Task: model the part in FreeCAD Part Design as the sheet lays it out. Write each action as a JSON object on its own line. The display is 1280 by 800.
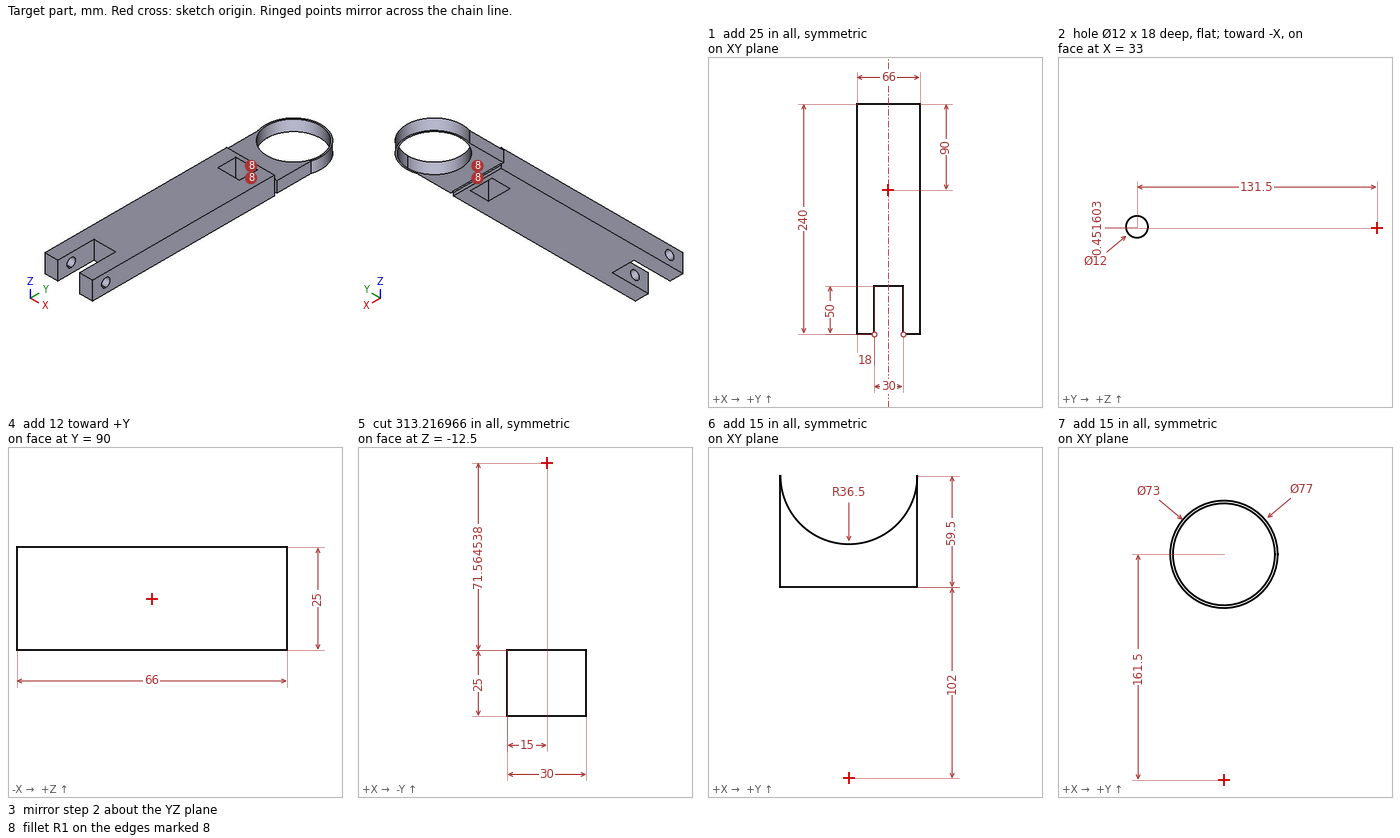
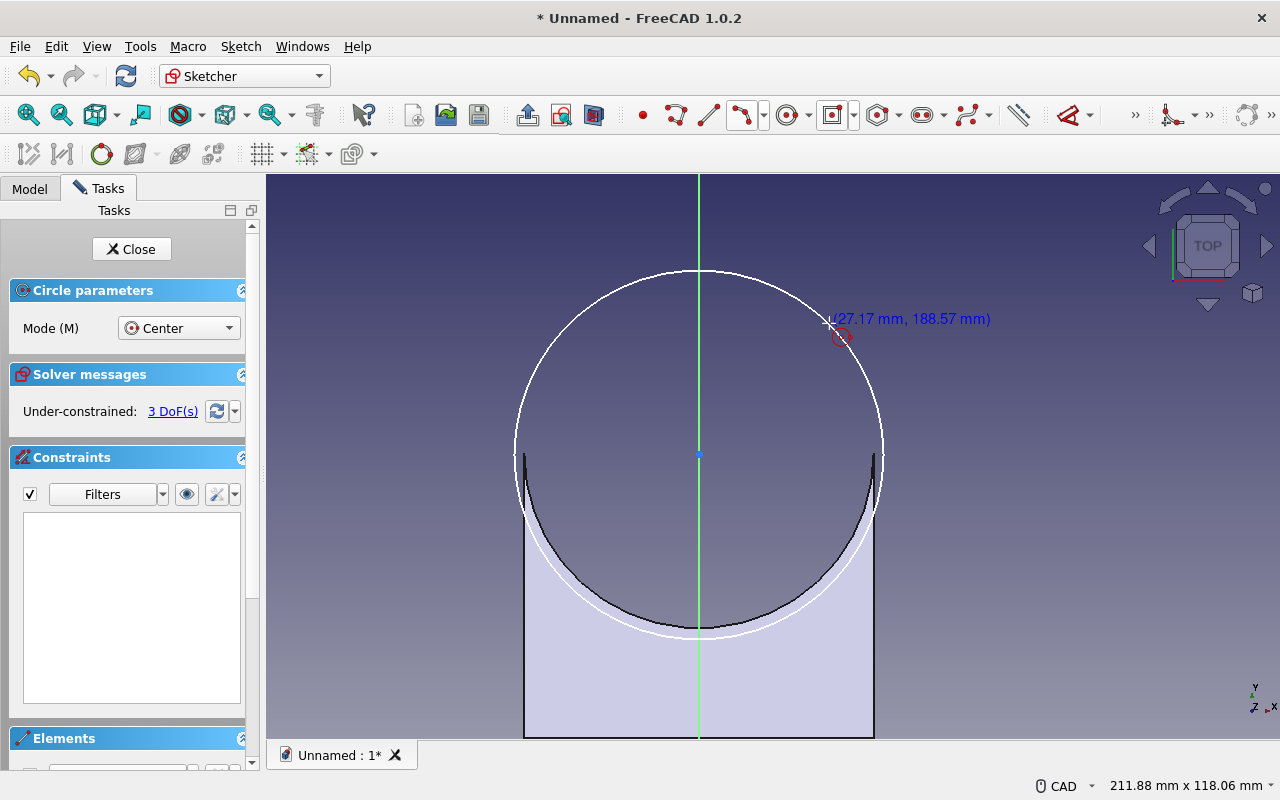
{"action": "left_click", "coordinate": [699, 455]}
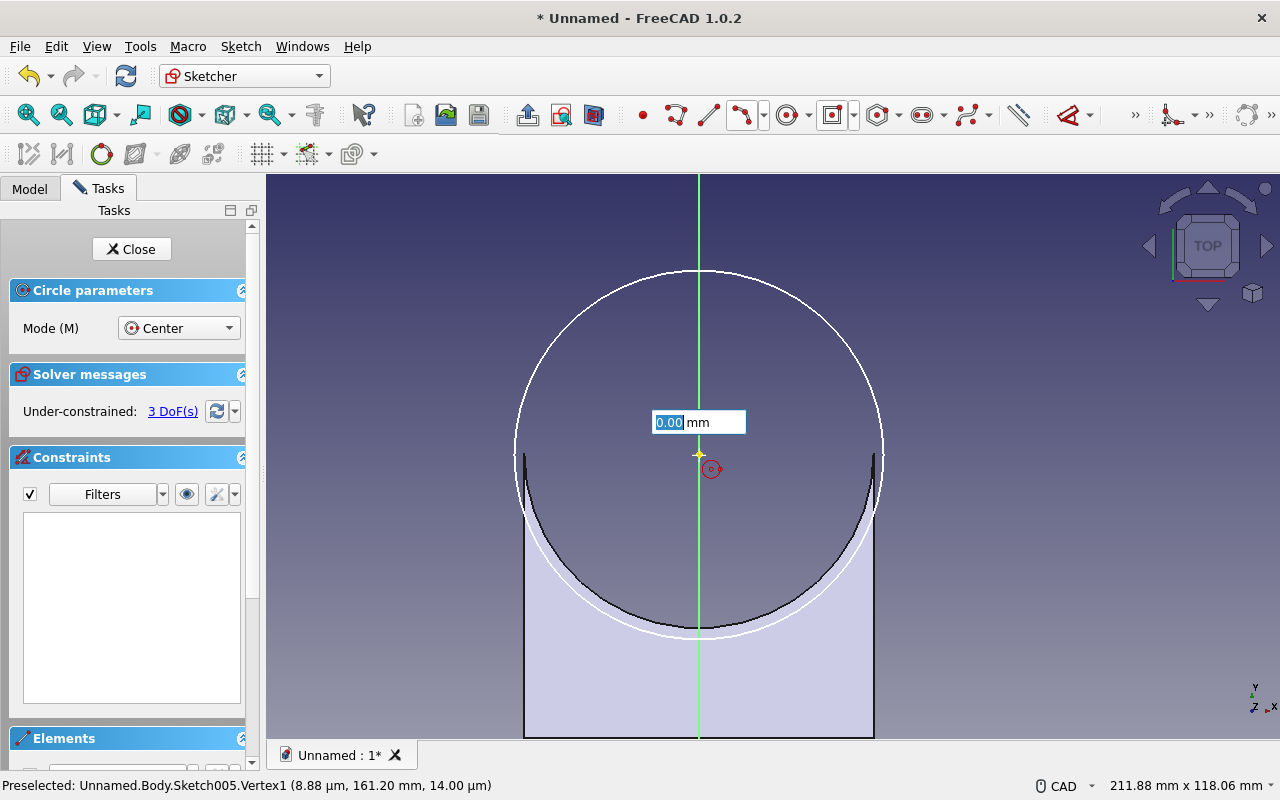
{"action": "scroll", "coordinate": [759, 289], "scroll_direction": "up", "scroll_amount": 3}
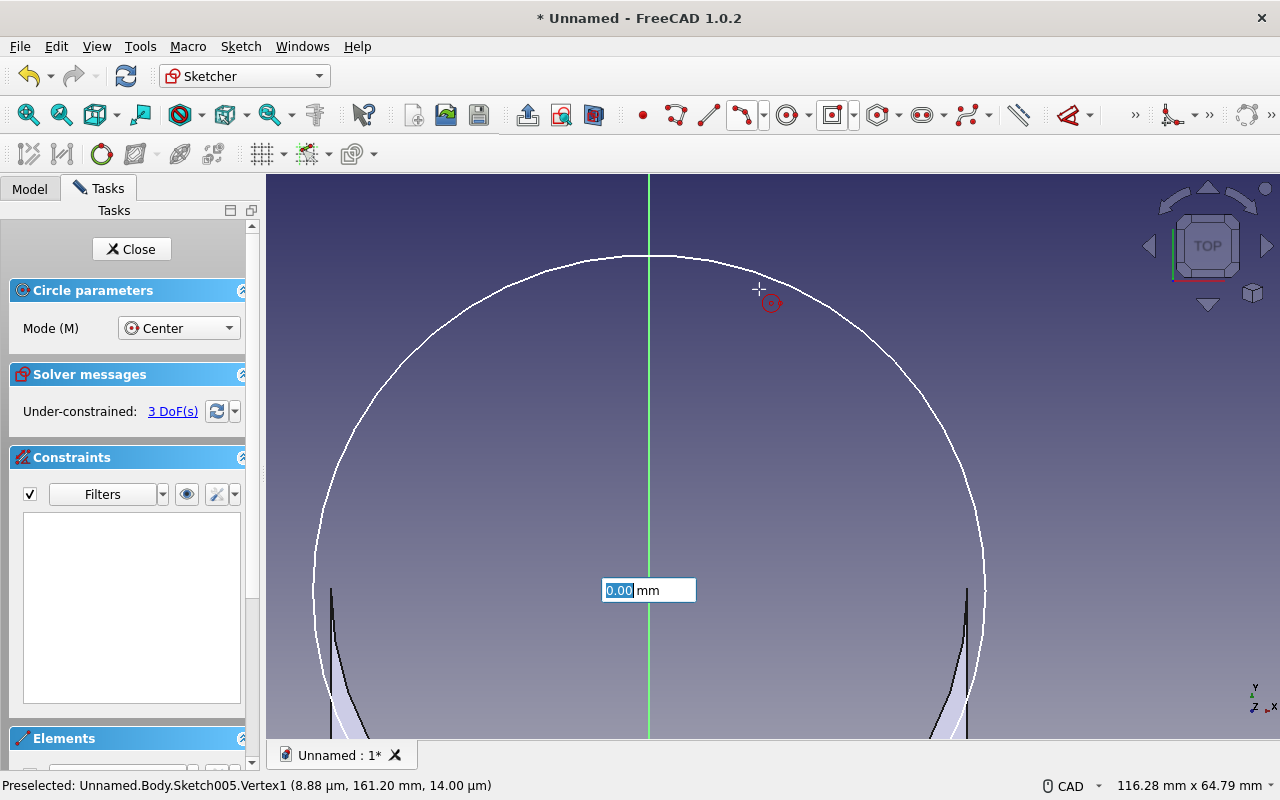
{"action": "left_click", "coordinate": [758, 290]}
{"action": "key", "text": "Escape"}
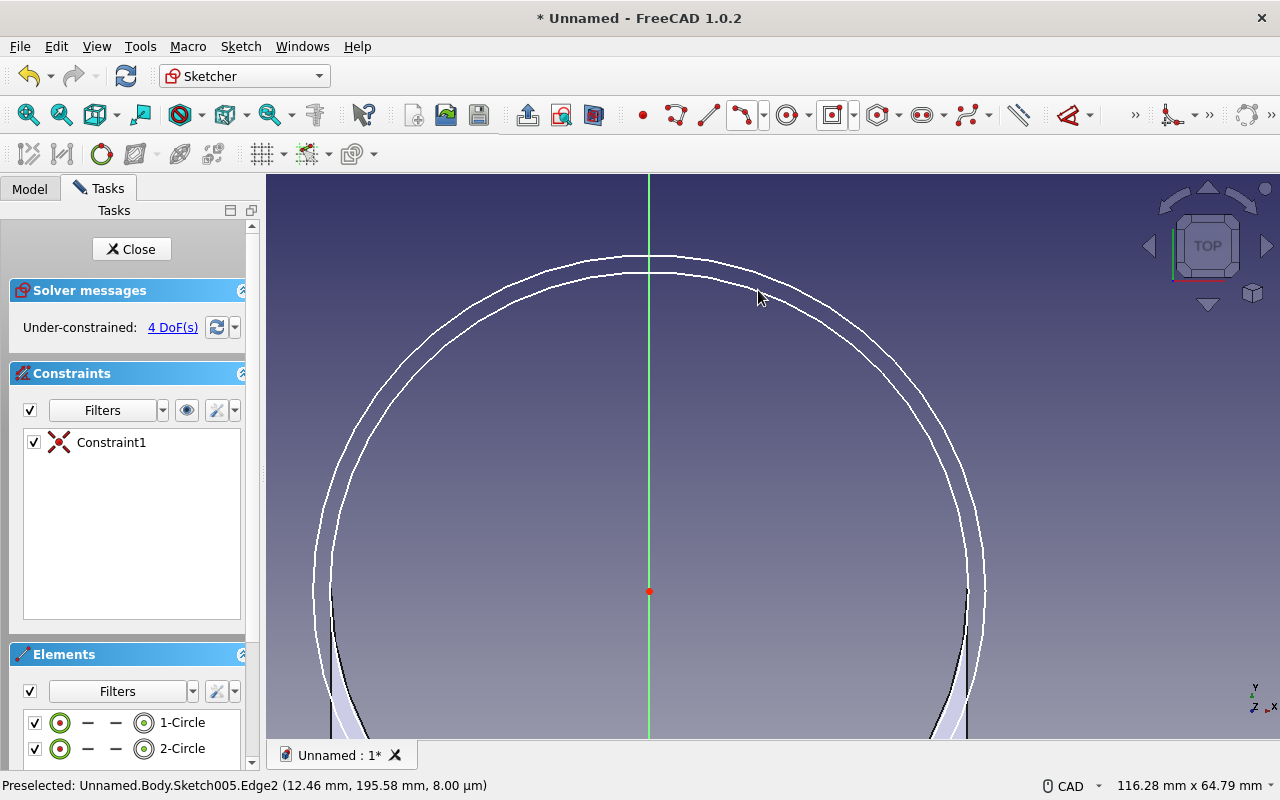
{"action": "left_click", "coordinate": [649, 591]}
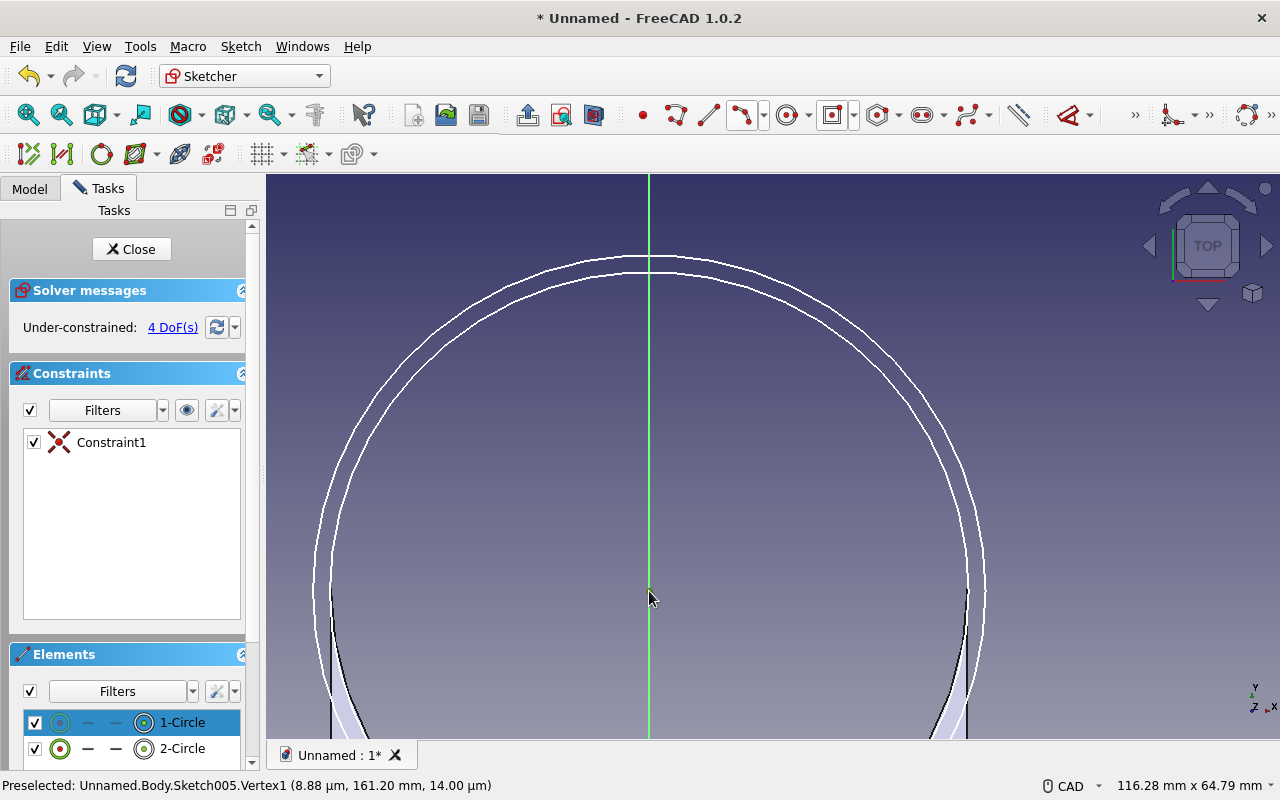
{"action": "left_click", "coordinate": [649, 675]}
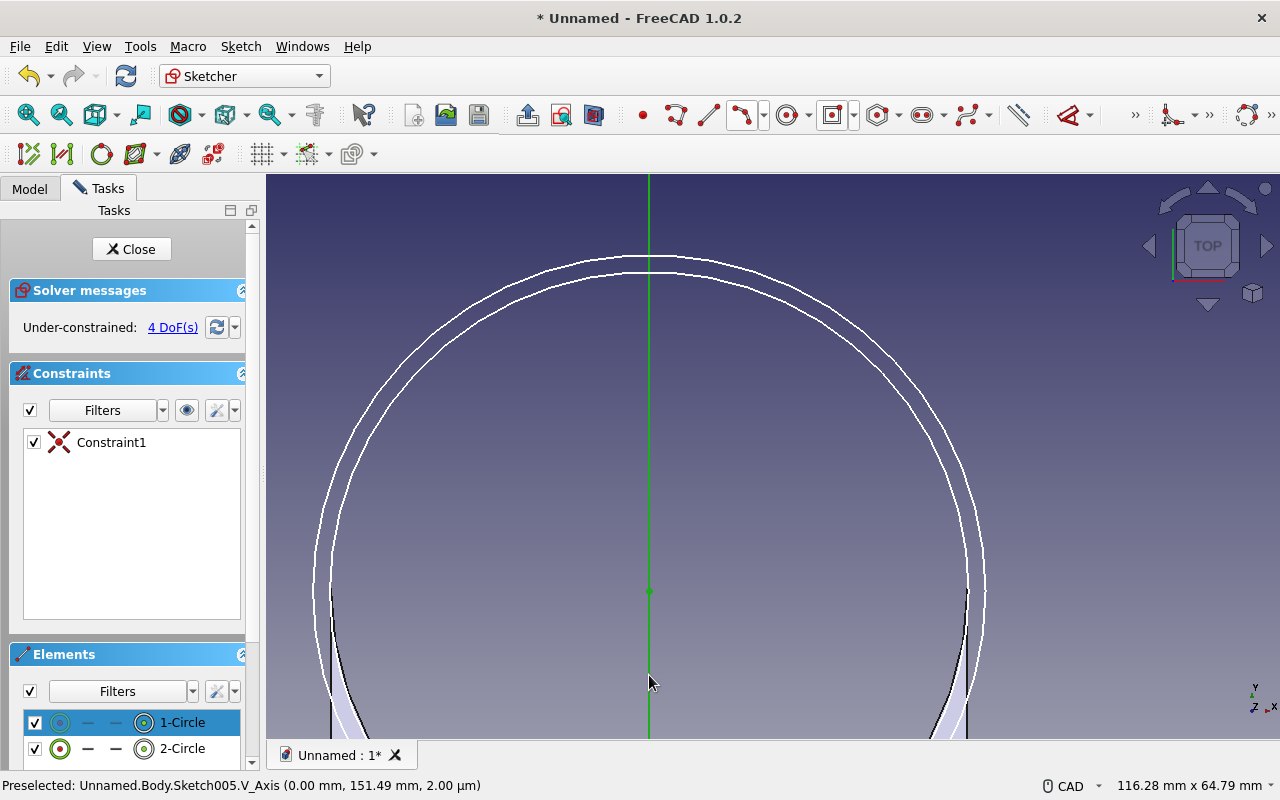
{"action": "key", "text": "c"}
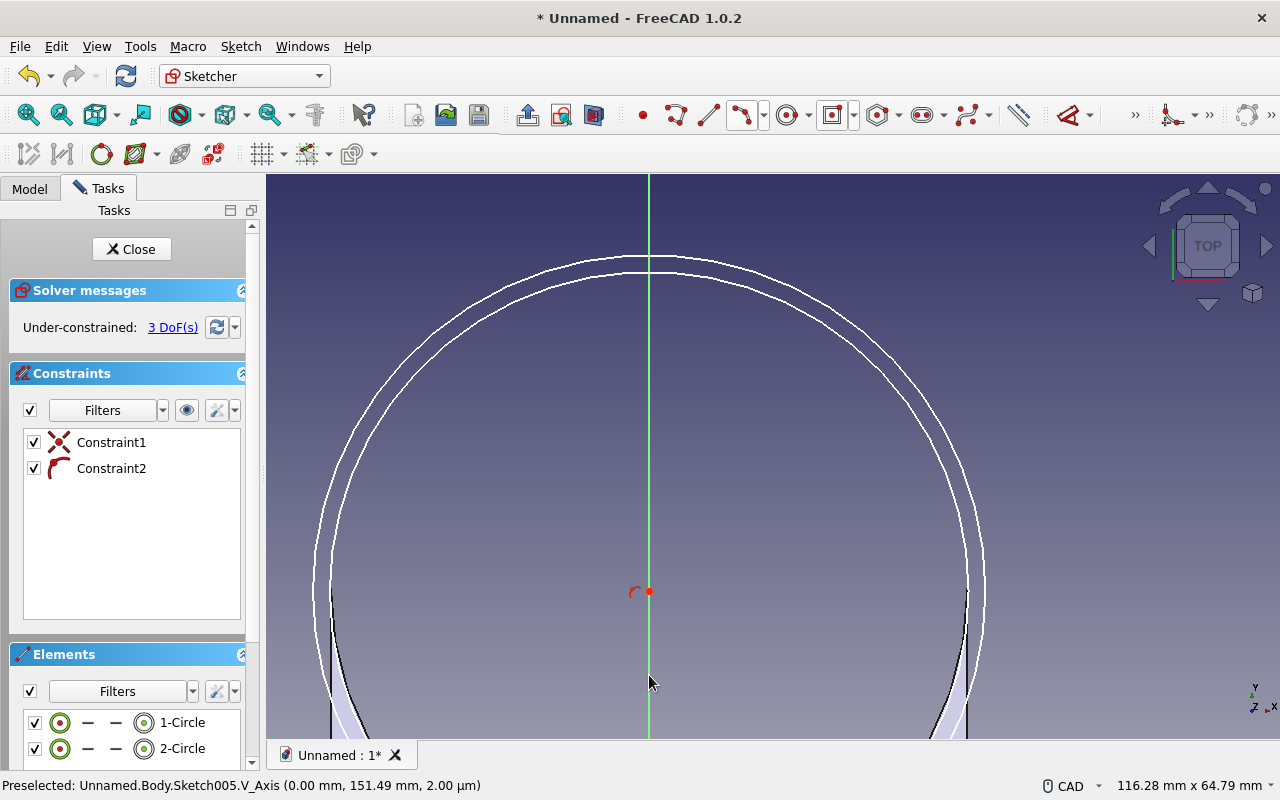
{"action": "key", "text": "d"}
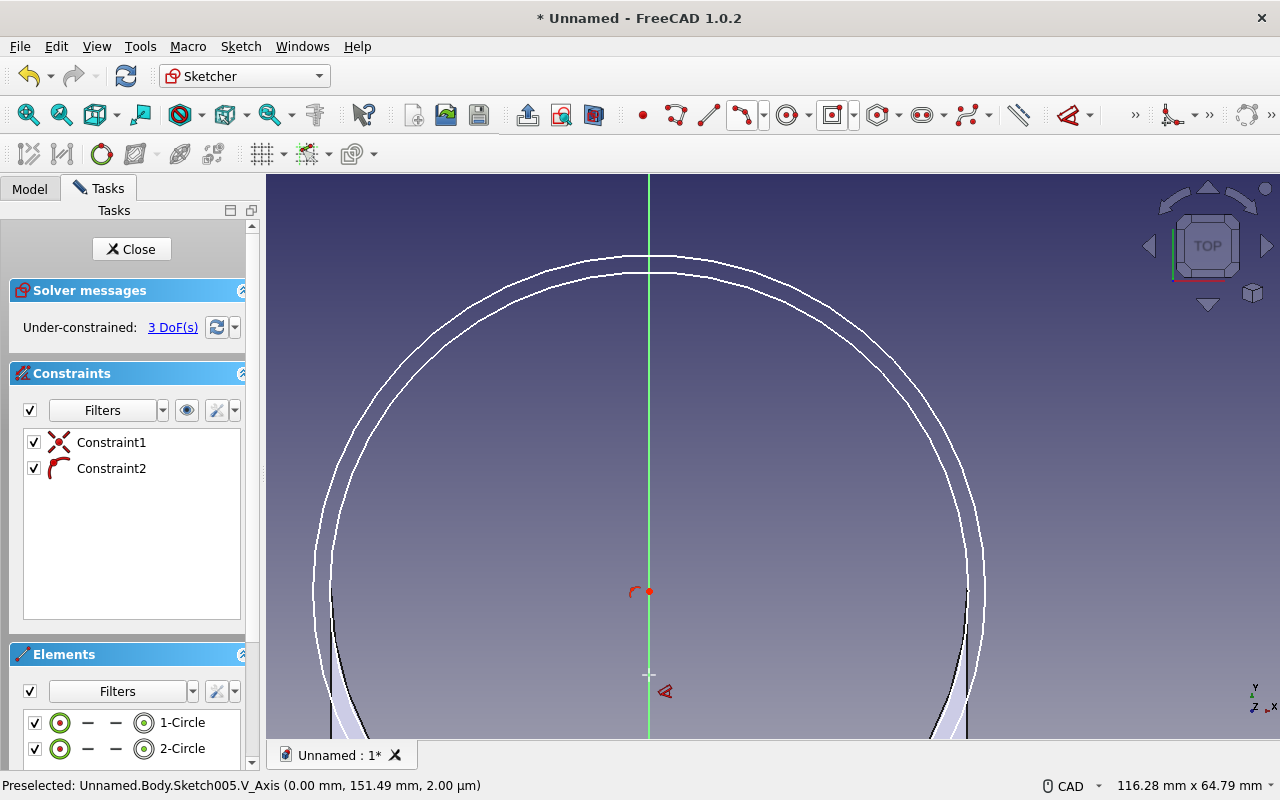
{"action": "left_click", "coordinate": [886, 353]}
{"action": "left_click", "coordinate": [909, 330]}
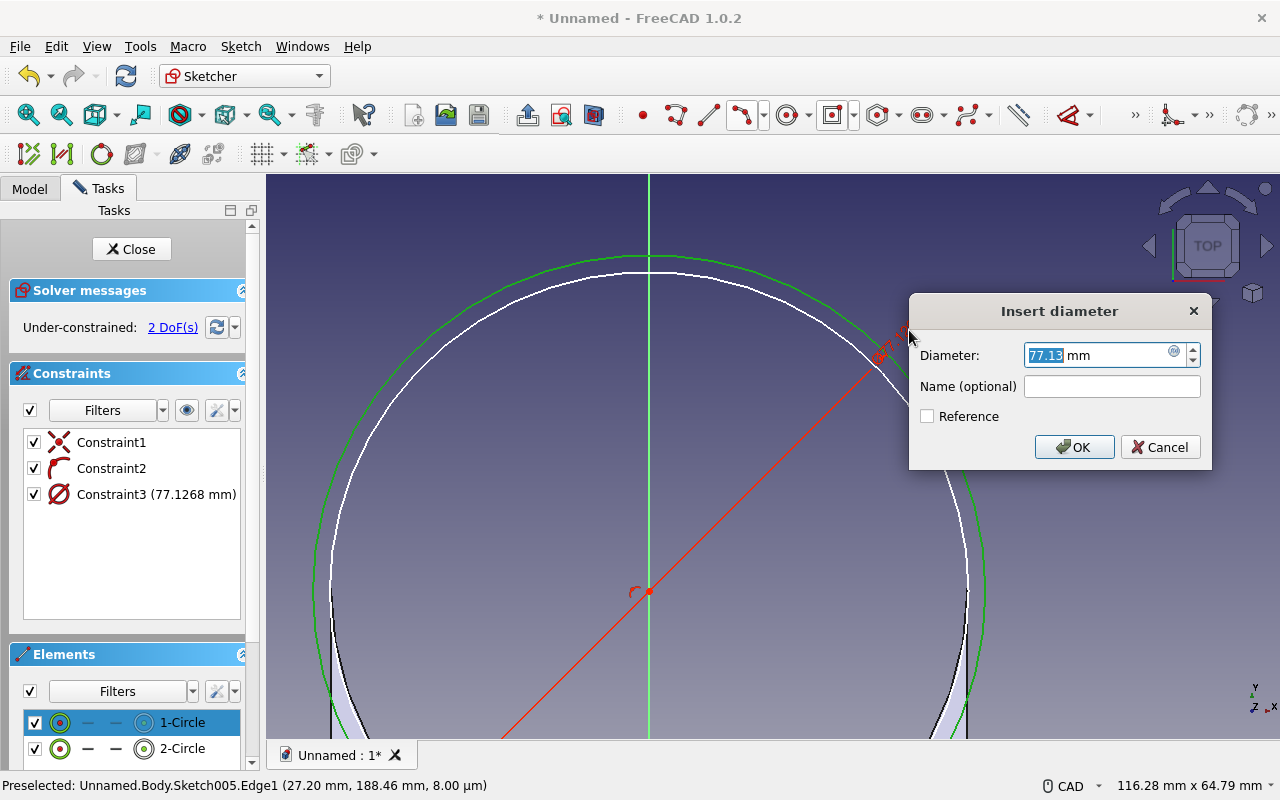
{"action": "type", "text": "77"}
{"action": "key", "text": "Return"}